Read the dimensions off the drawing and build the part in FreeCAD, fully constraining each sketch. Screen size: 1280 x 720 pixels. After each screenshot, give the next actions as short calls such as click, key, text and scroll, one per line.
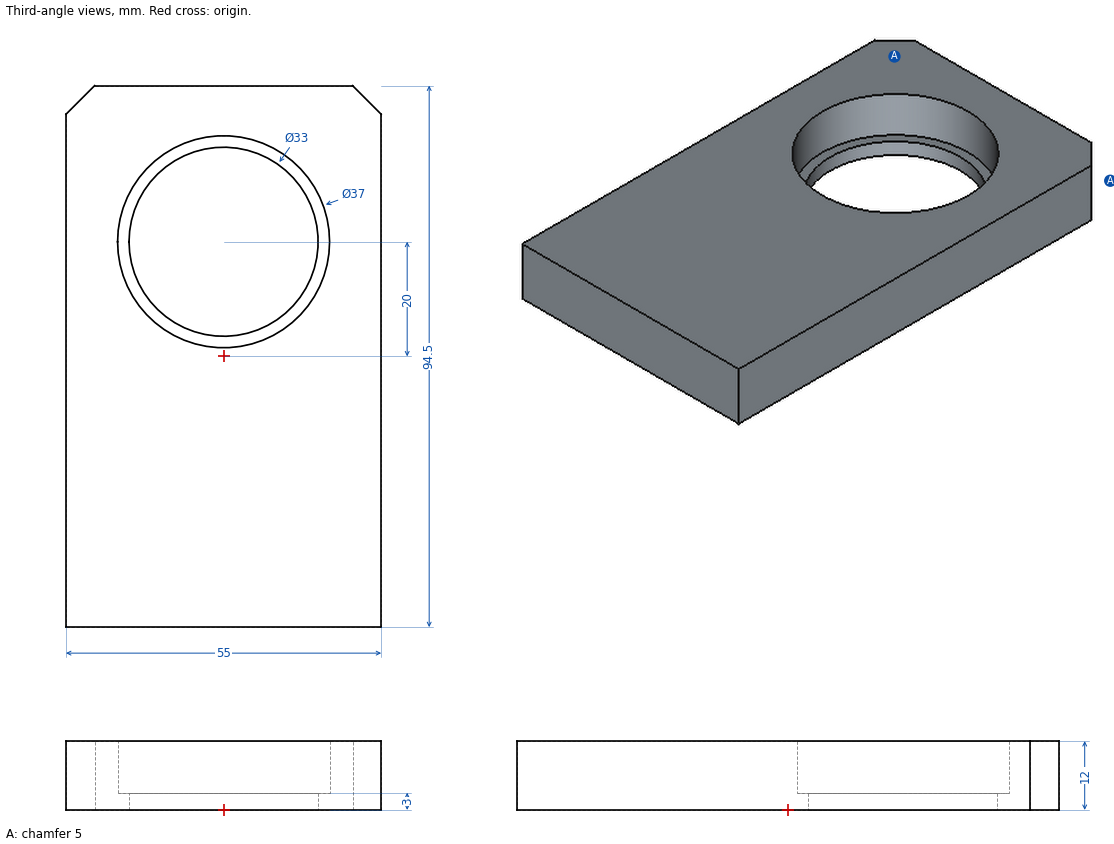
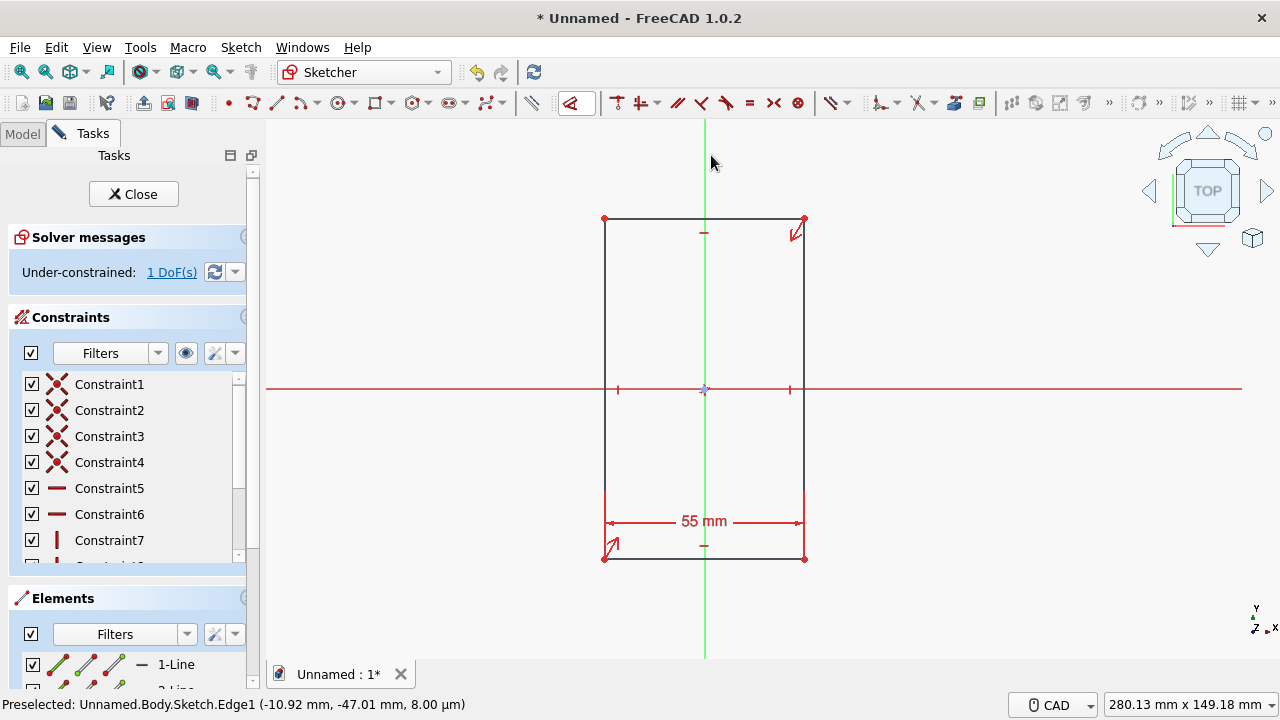
click(804, 457)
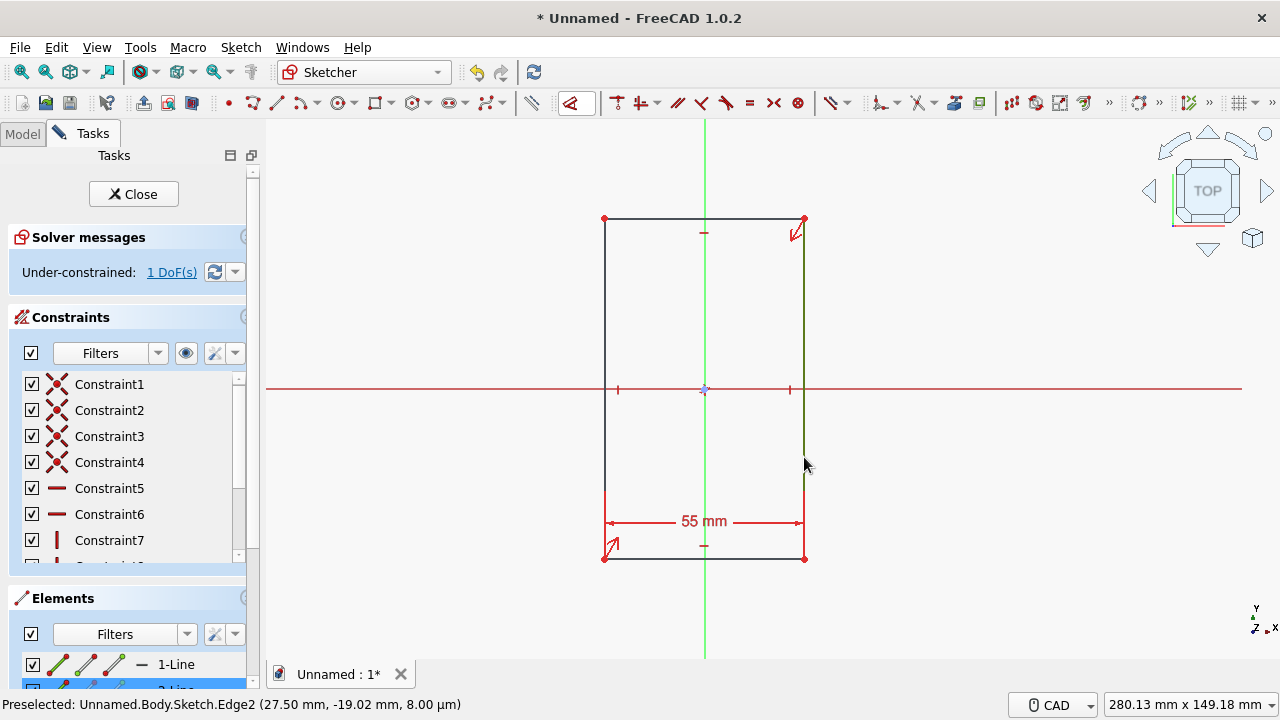
click(590, 104)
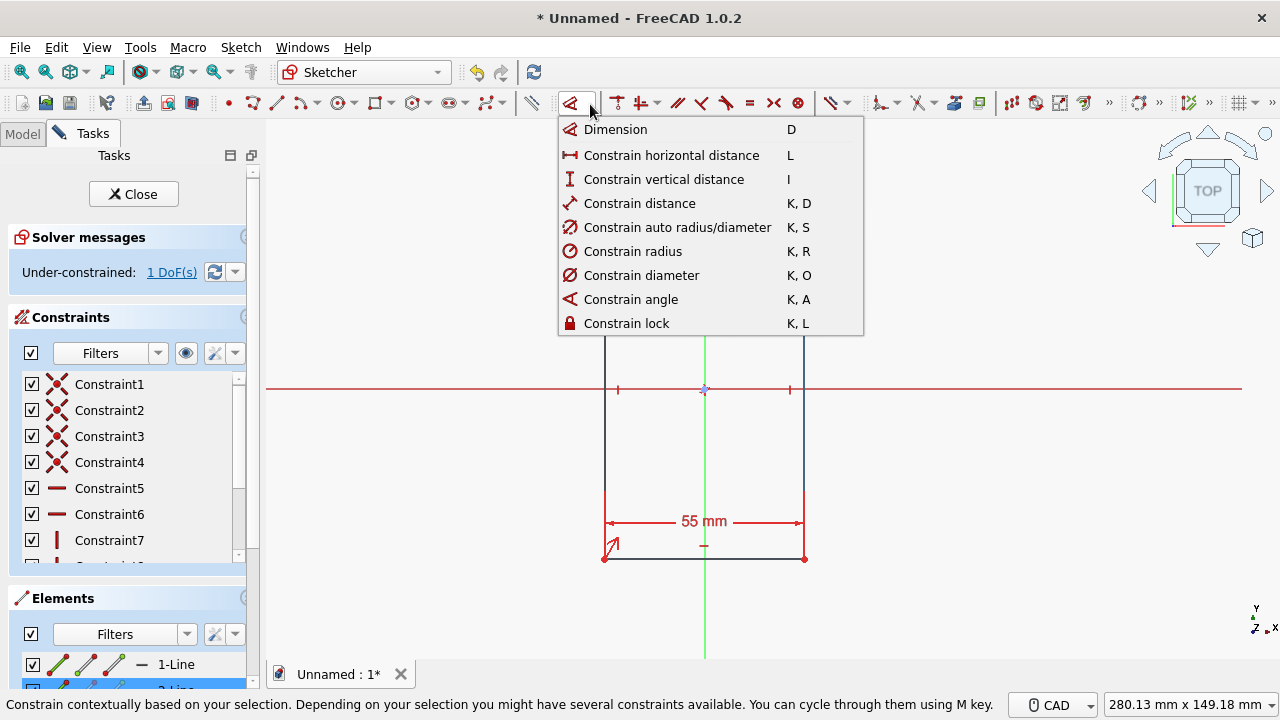
click(711, 179)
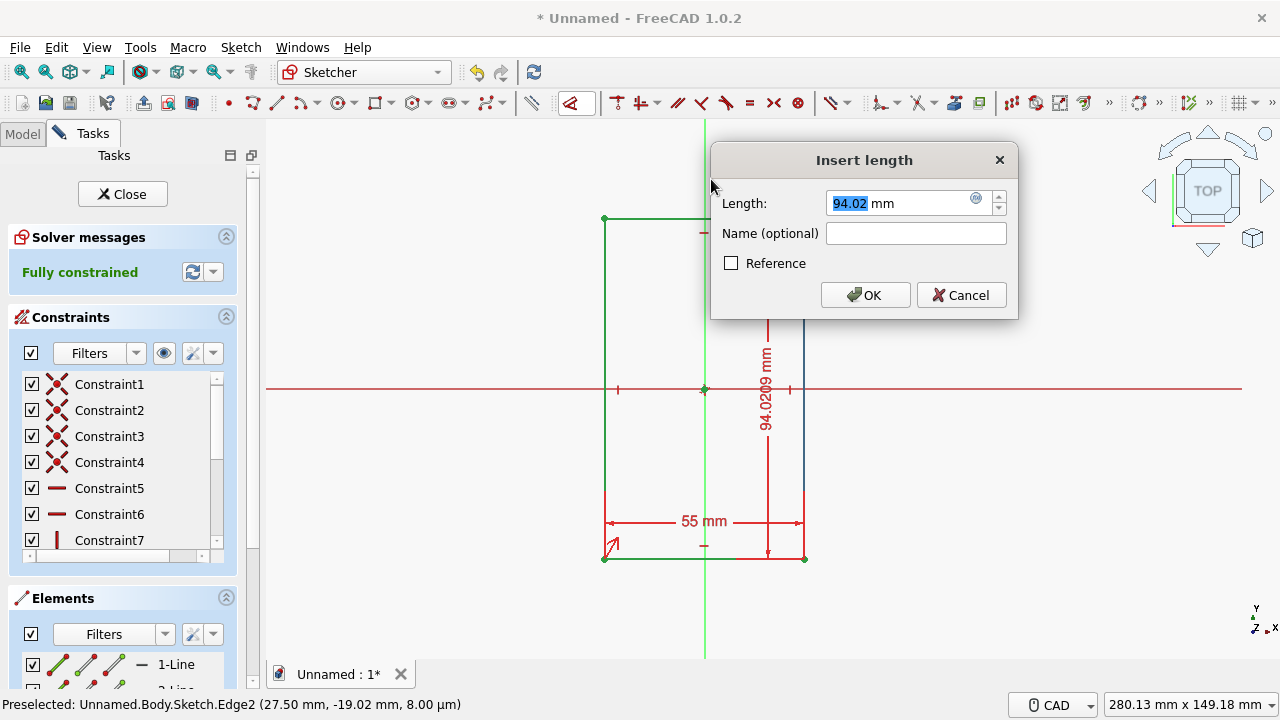
text(94.5)
key(Return)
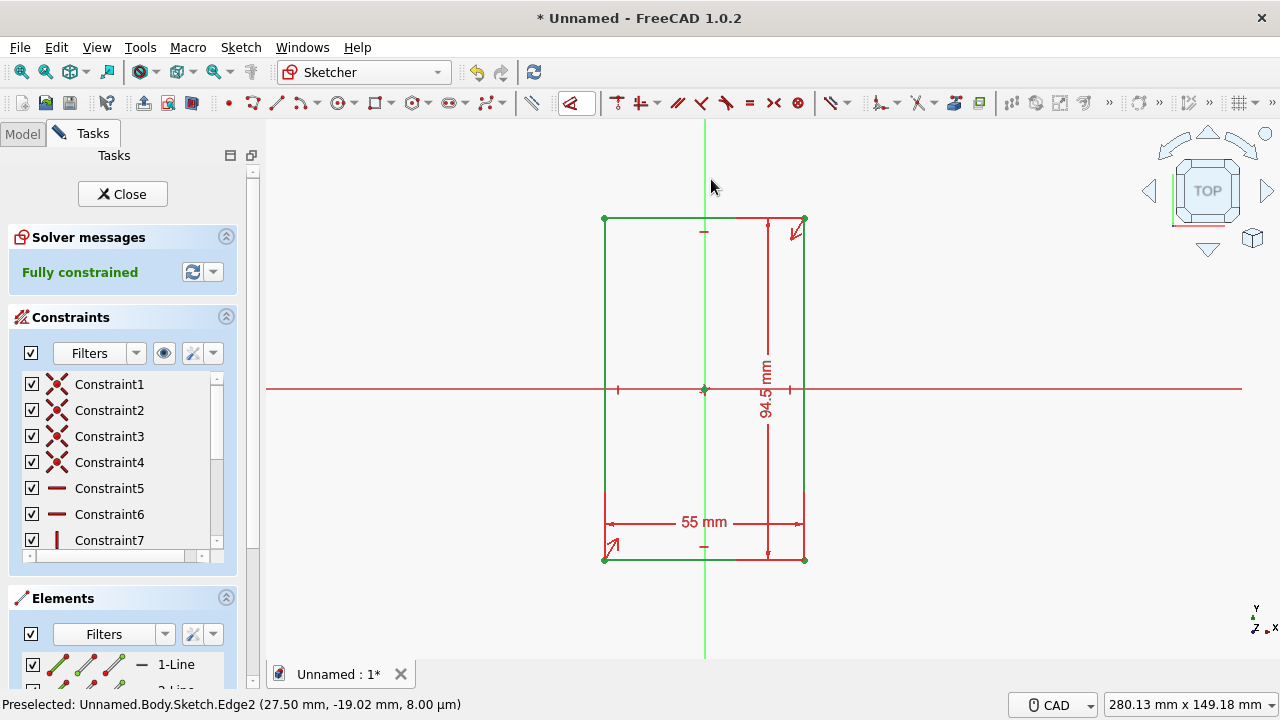
click(123, 194)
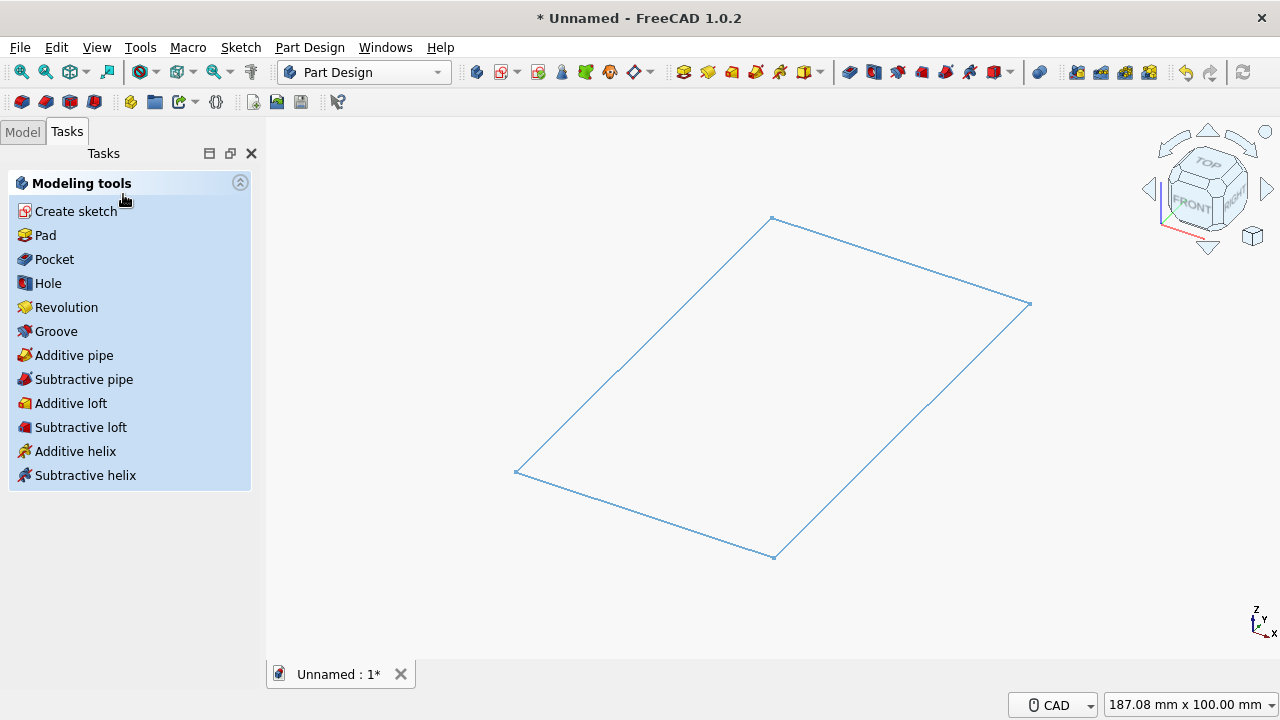
click(684, 72)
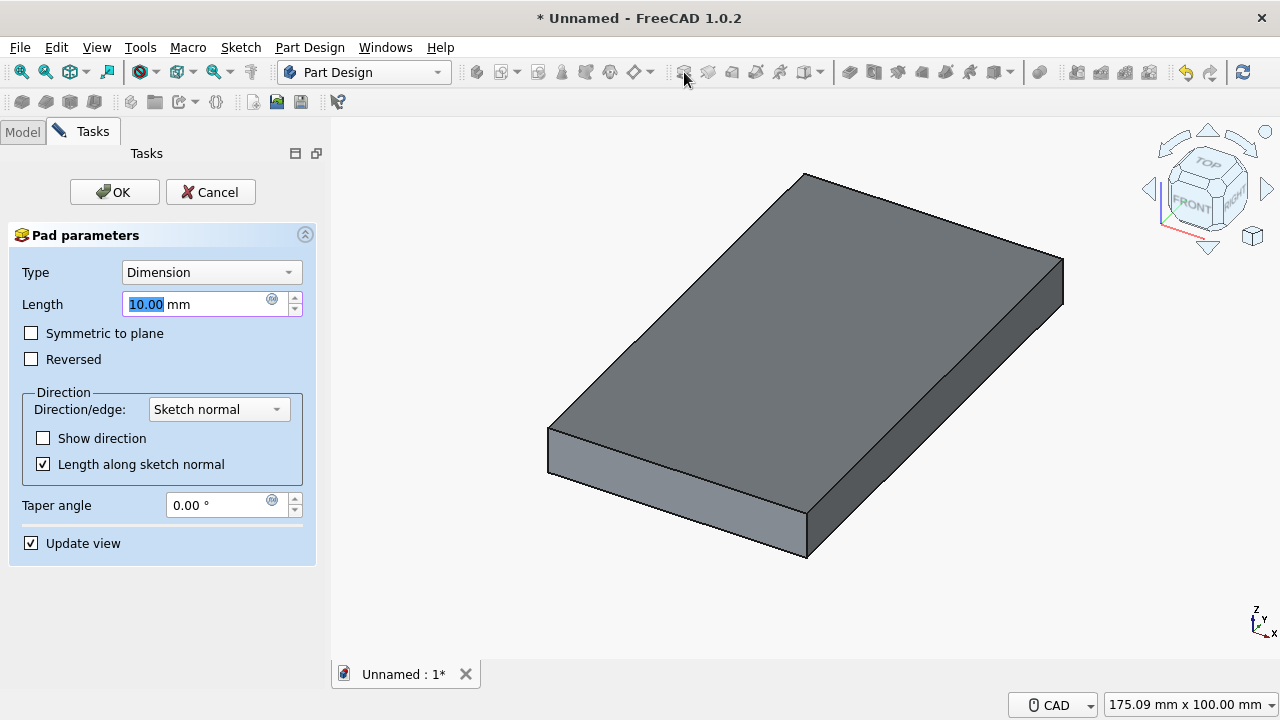
text(12)
key(Tab)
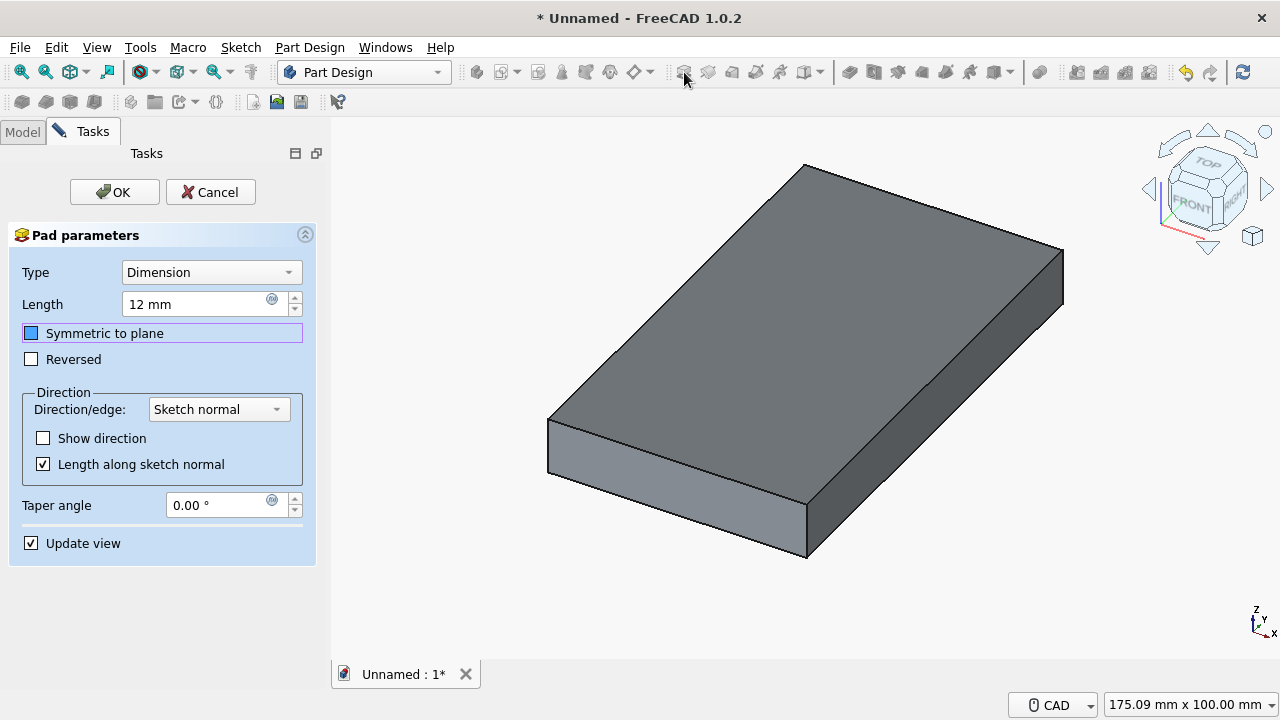
click(115, 192)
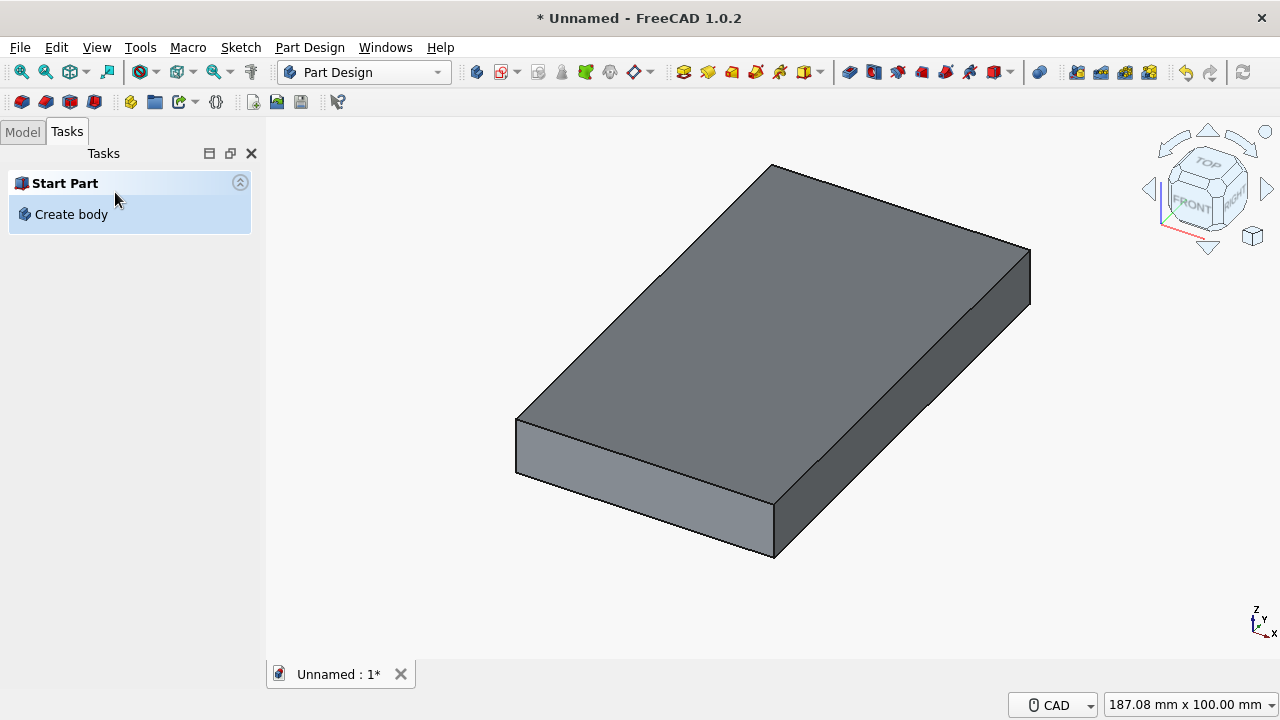
key(5)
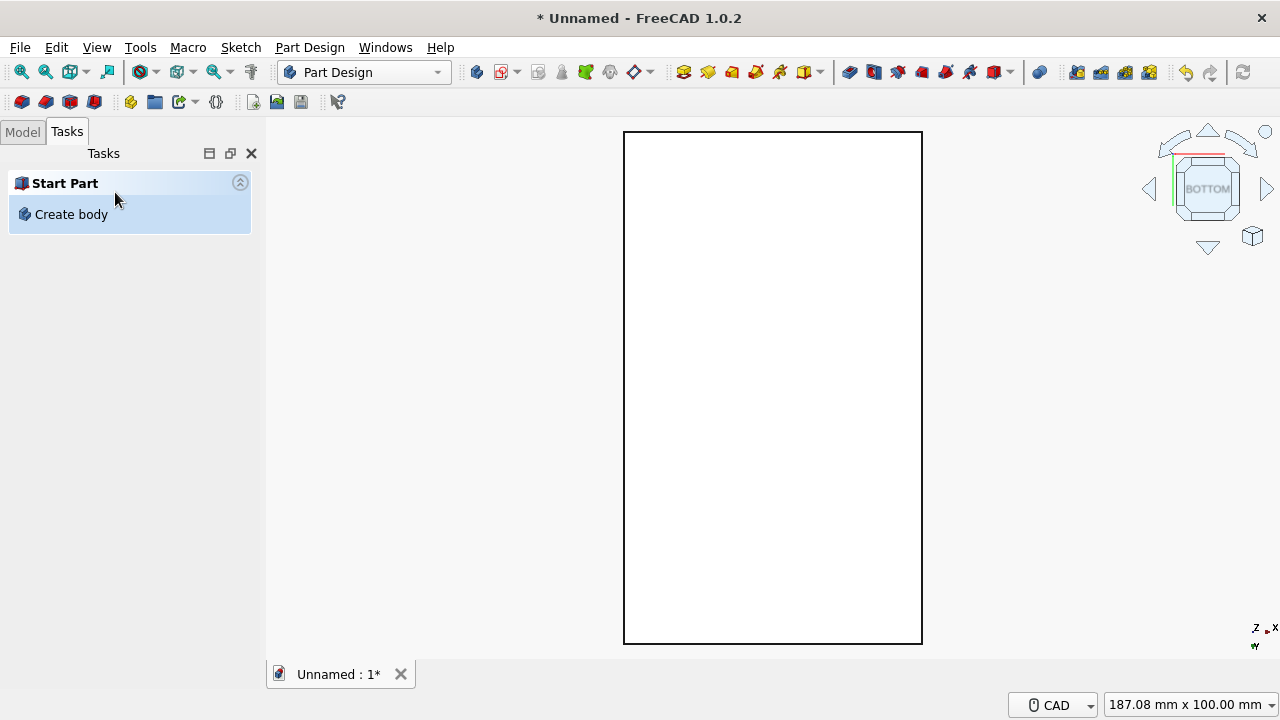
click(773, 460)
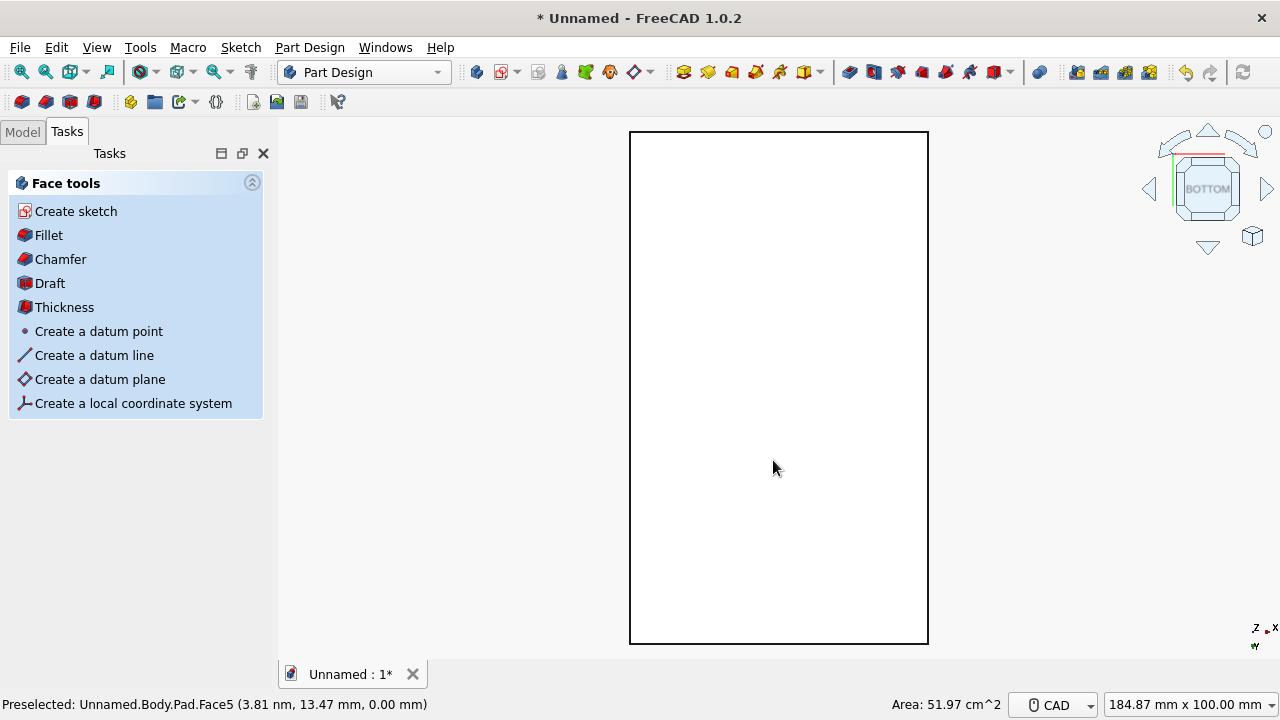
click(502, 72)